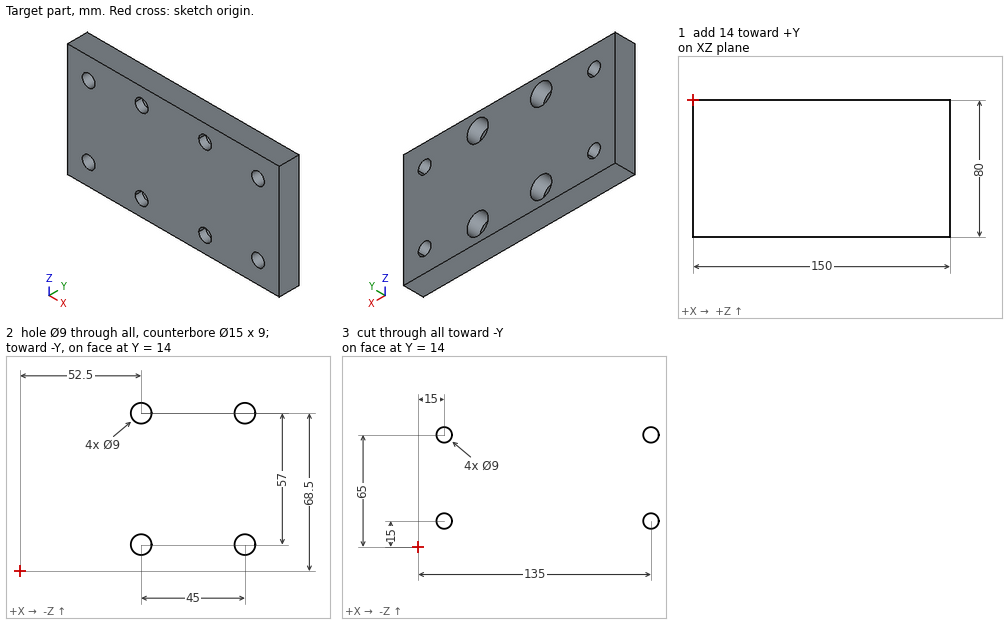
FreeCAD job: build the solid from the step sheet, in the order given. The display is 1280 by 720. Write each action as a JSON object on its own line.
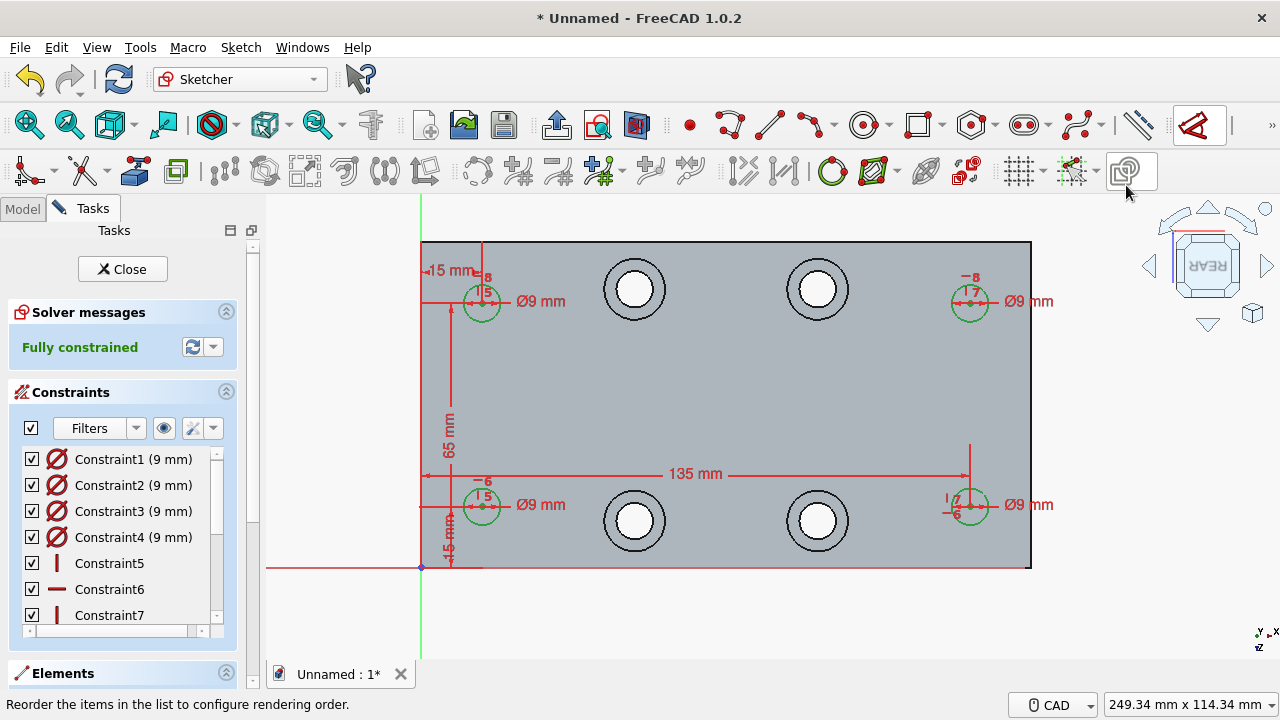
{"action": "left_click", "coordinate": [123, 269]}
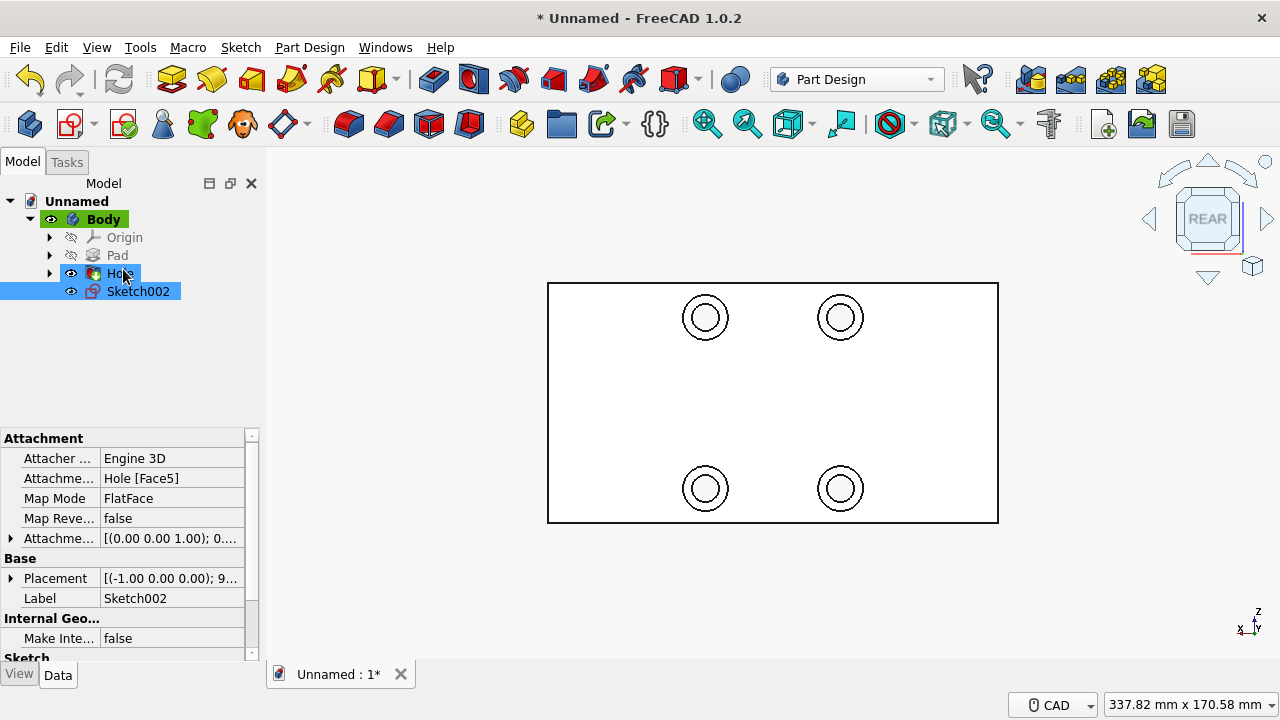
{"action": "left_click", "coordinate": [434, 80]}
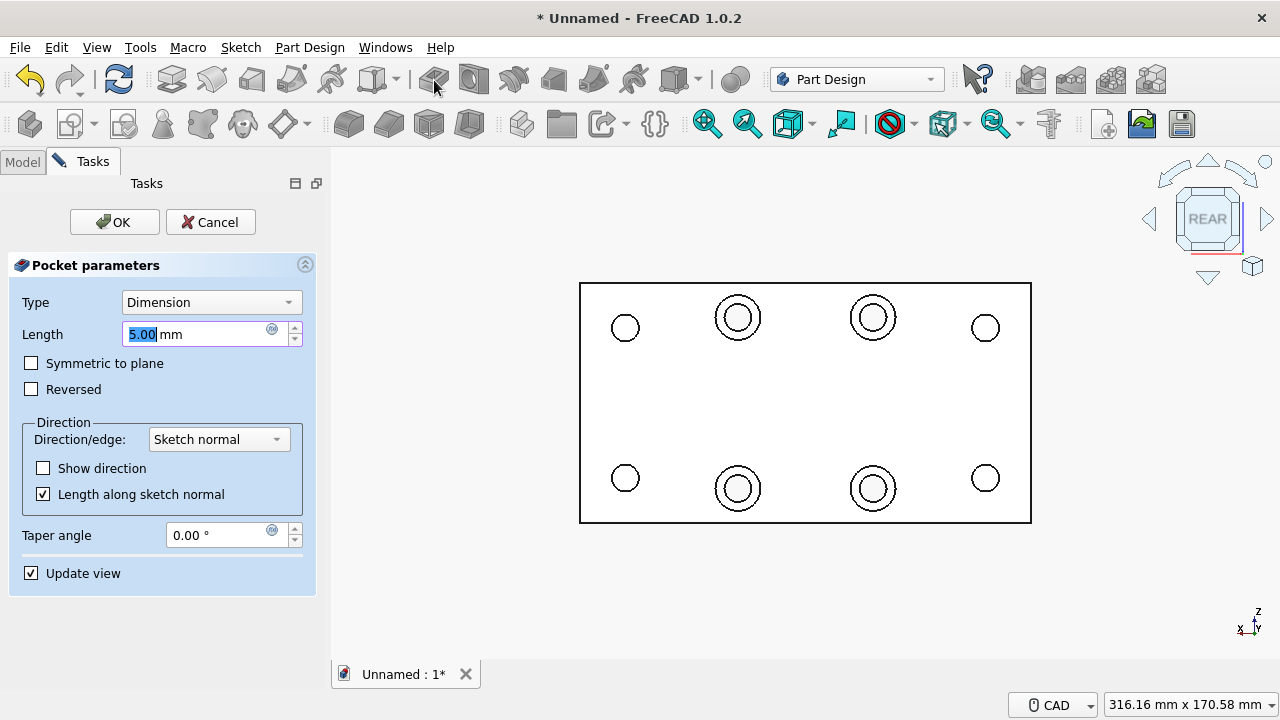
{"action": "left_click", "coordinate": [212, 302]}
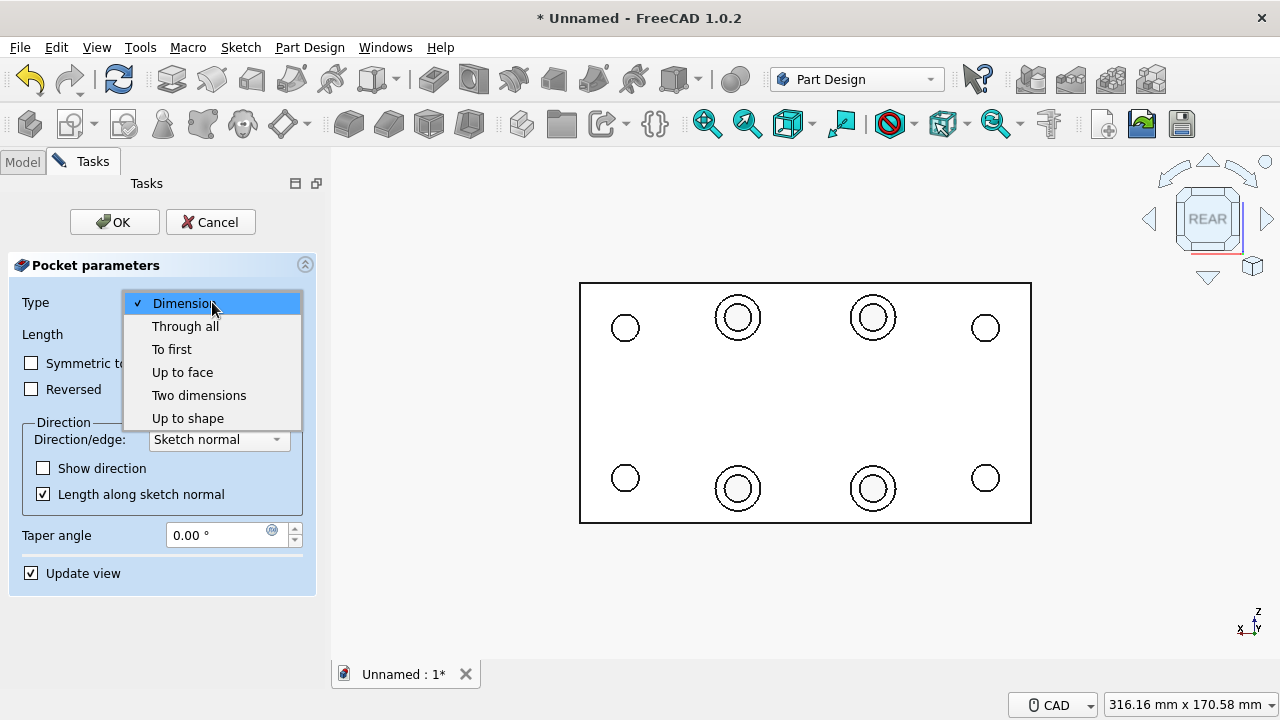
{"action": "left_click", "coordinate": [212, 326]}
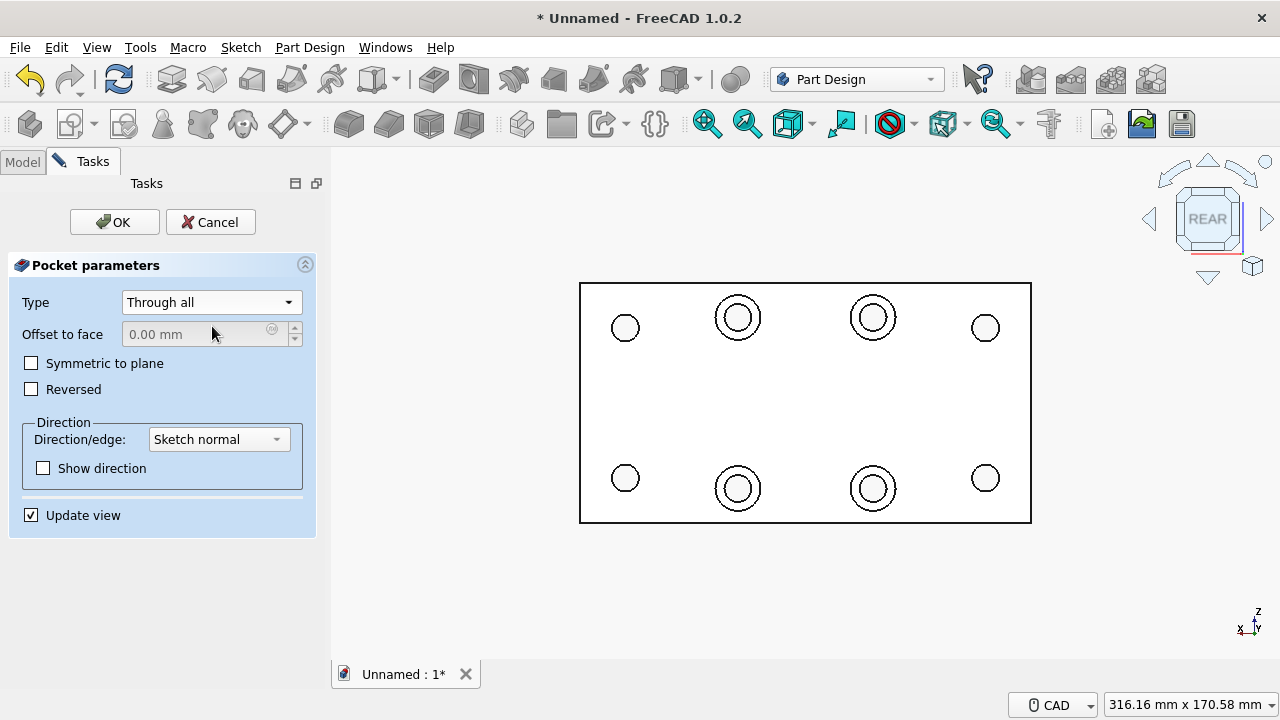
{"action": "left_click", "coordinate": [115, 222]}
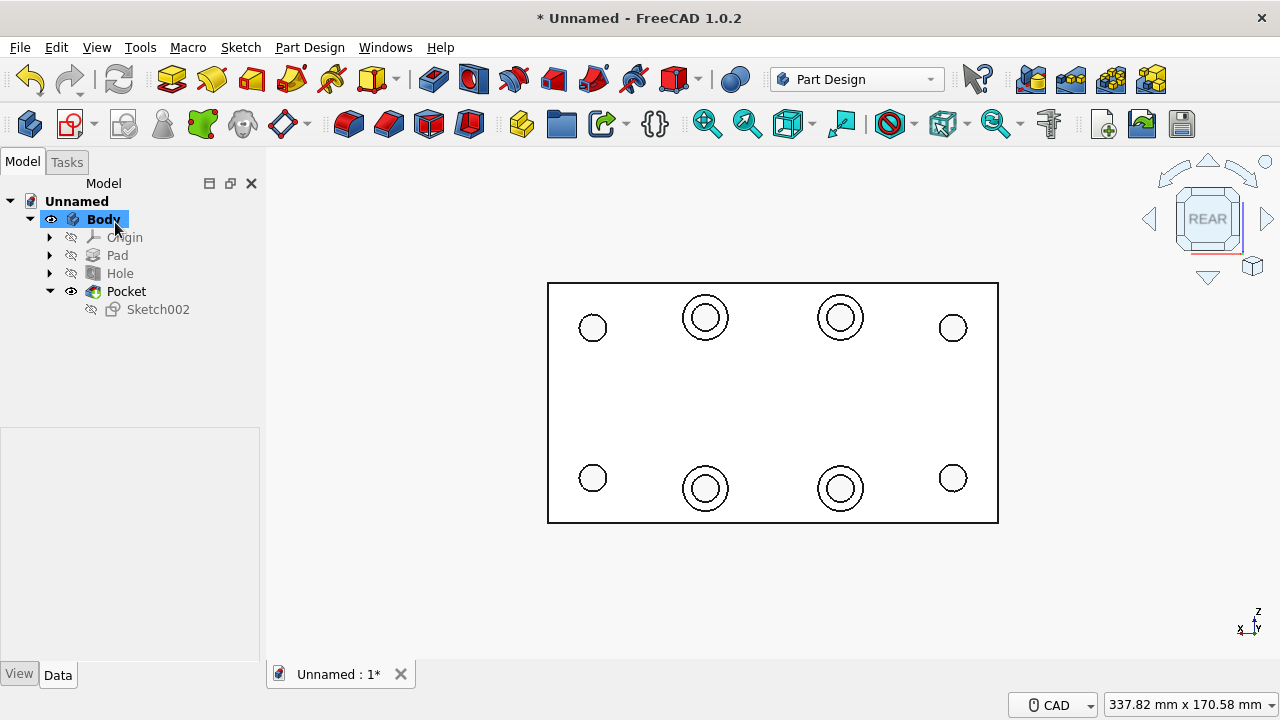
{"action": "key", "text": "0"}